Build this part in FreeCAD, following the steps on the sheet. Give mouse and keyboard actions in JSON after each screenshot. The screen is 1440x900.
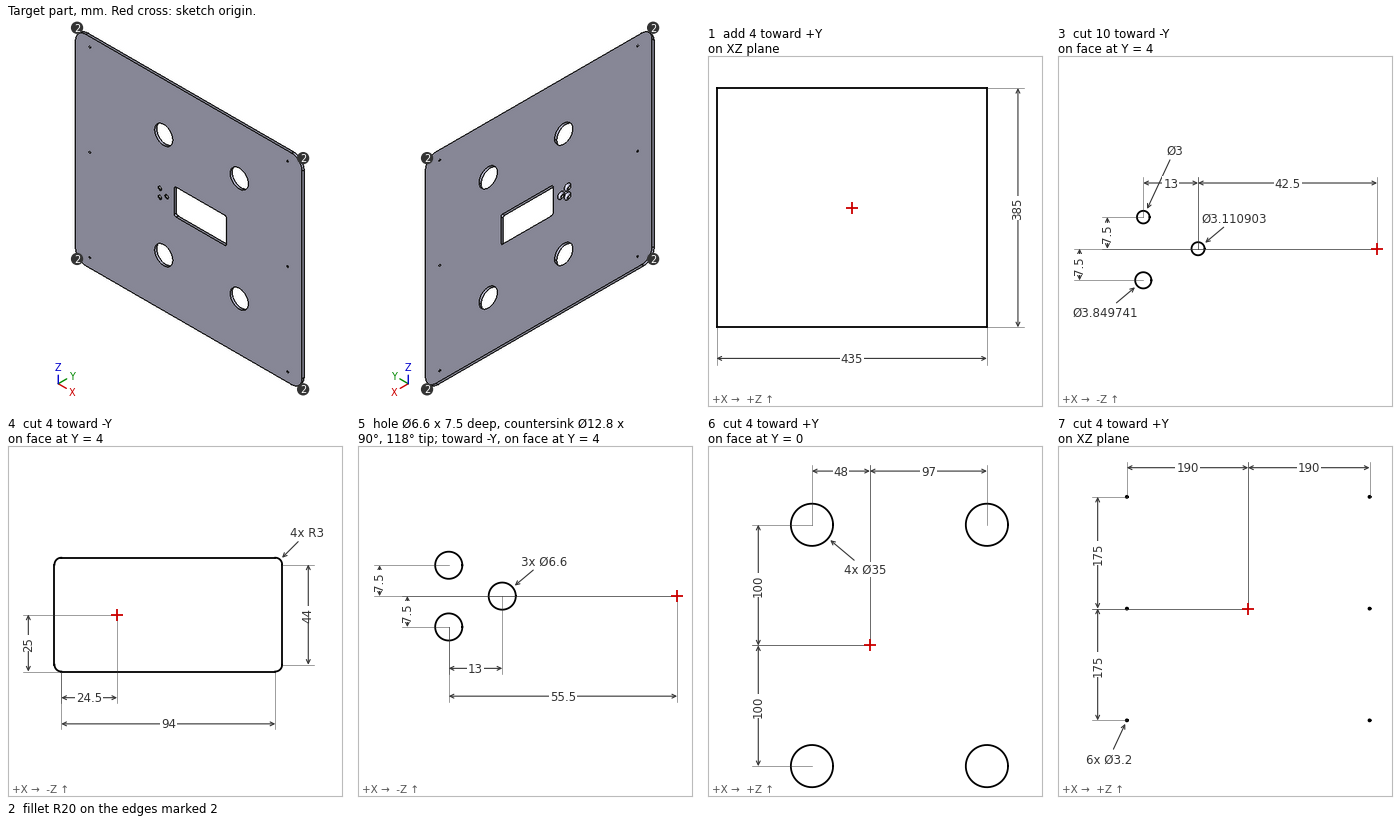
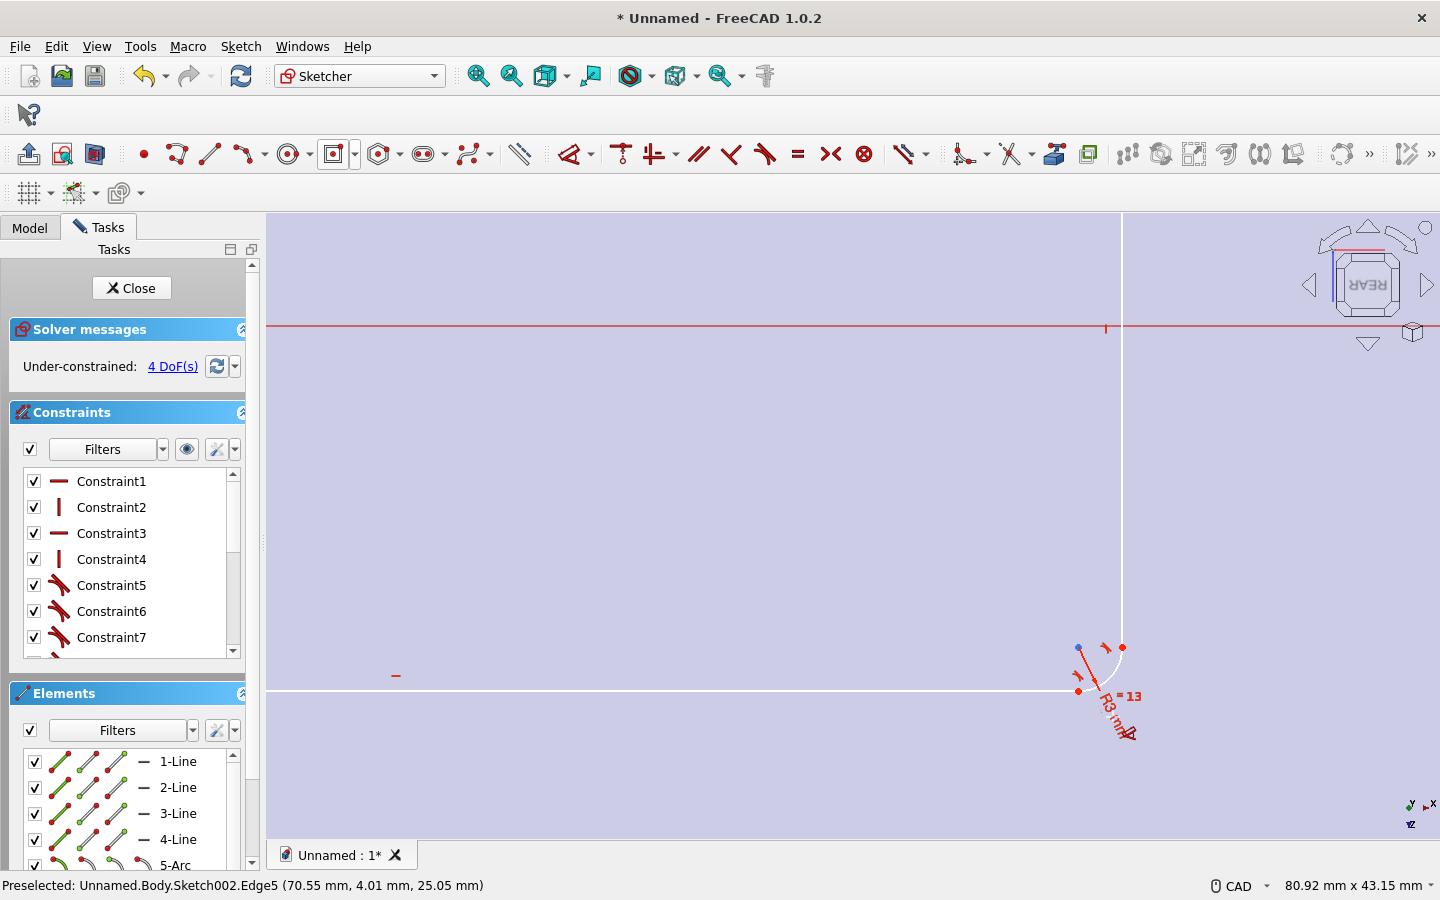
{"action": "left_click", "coordinate": [670, 691]}
{"action": "left_click", "coordinate": [686, 725]}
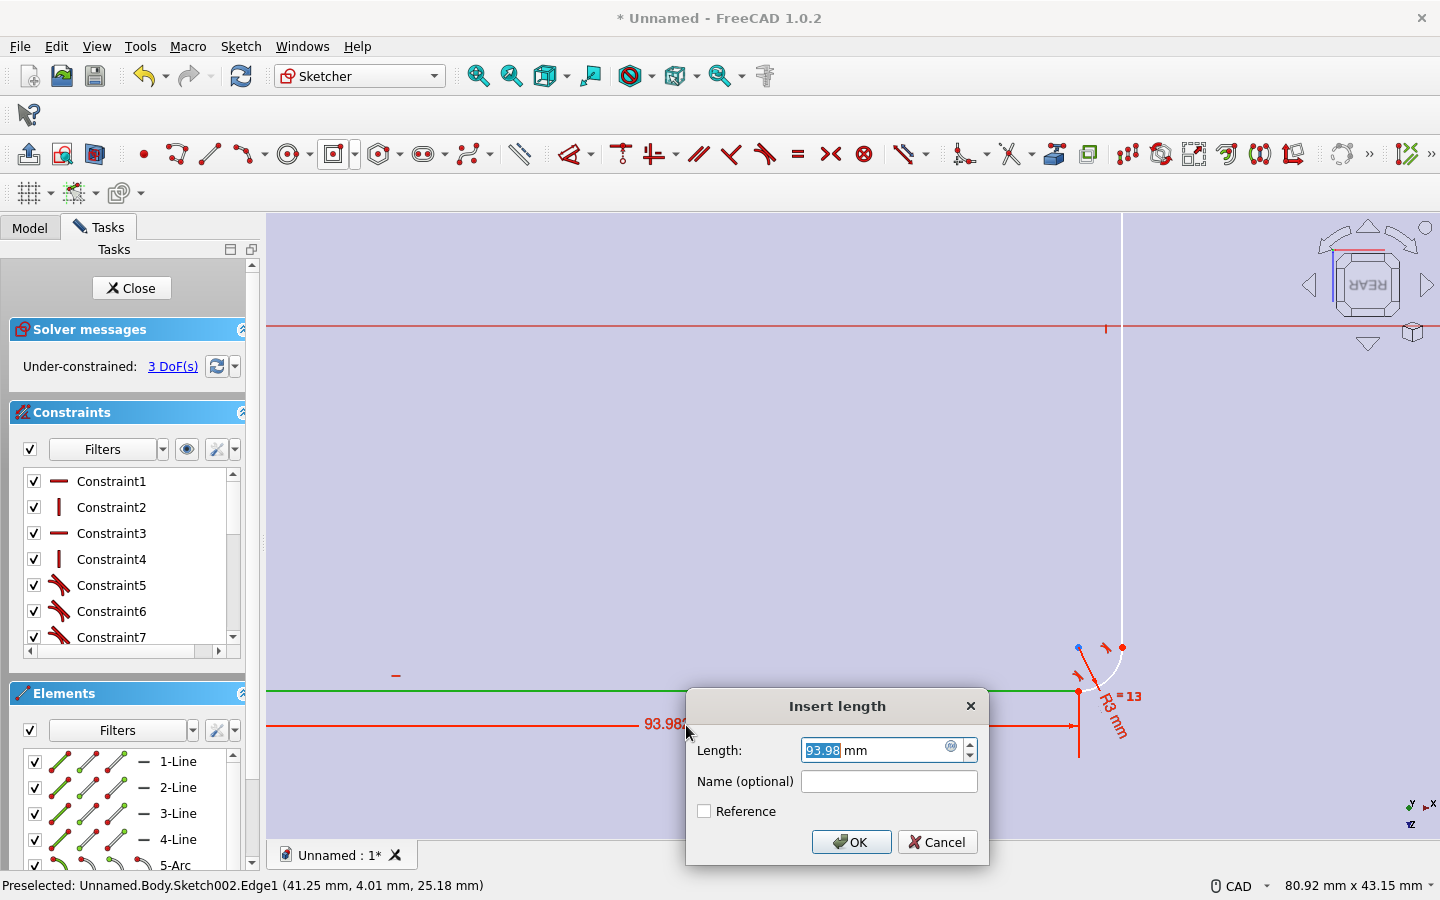
{"action": "type", "text": "94"}
{"action": "key", "text": "Return"}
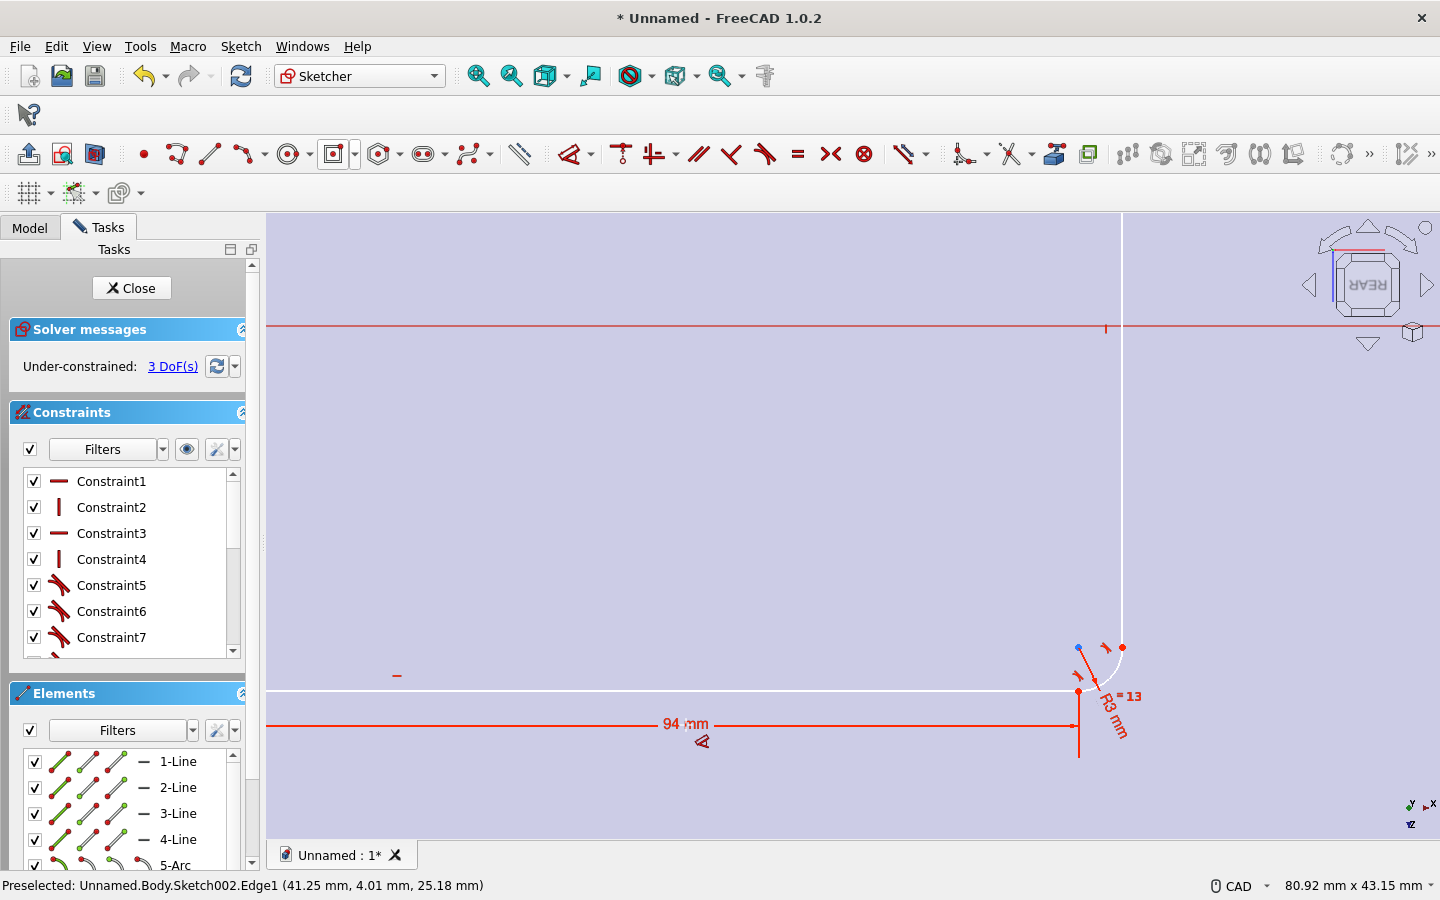
{"action": "left_click", "coordinate": [1122, 456]}
{"action": "left_click", "coordinate": [1156, 444]}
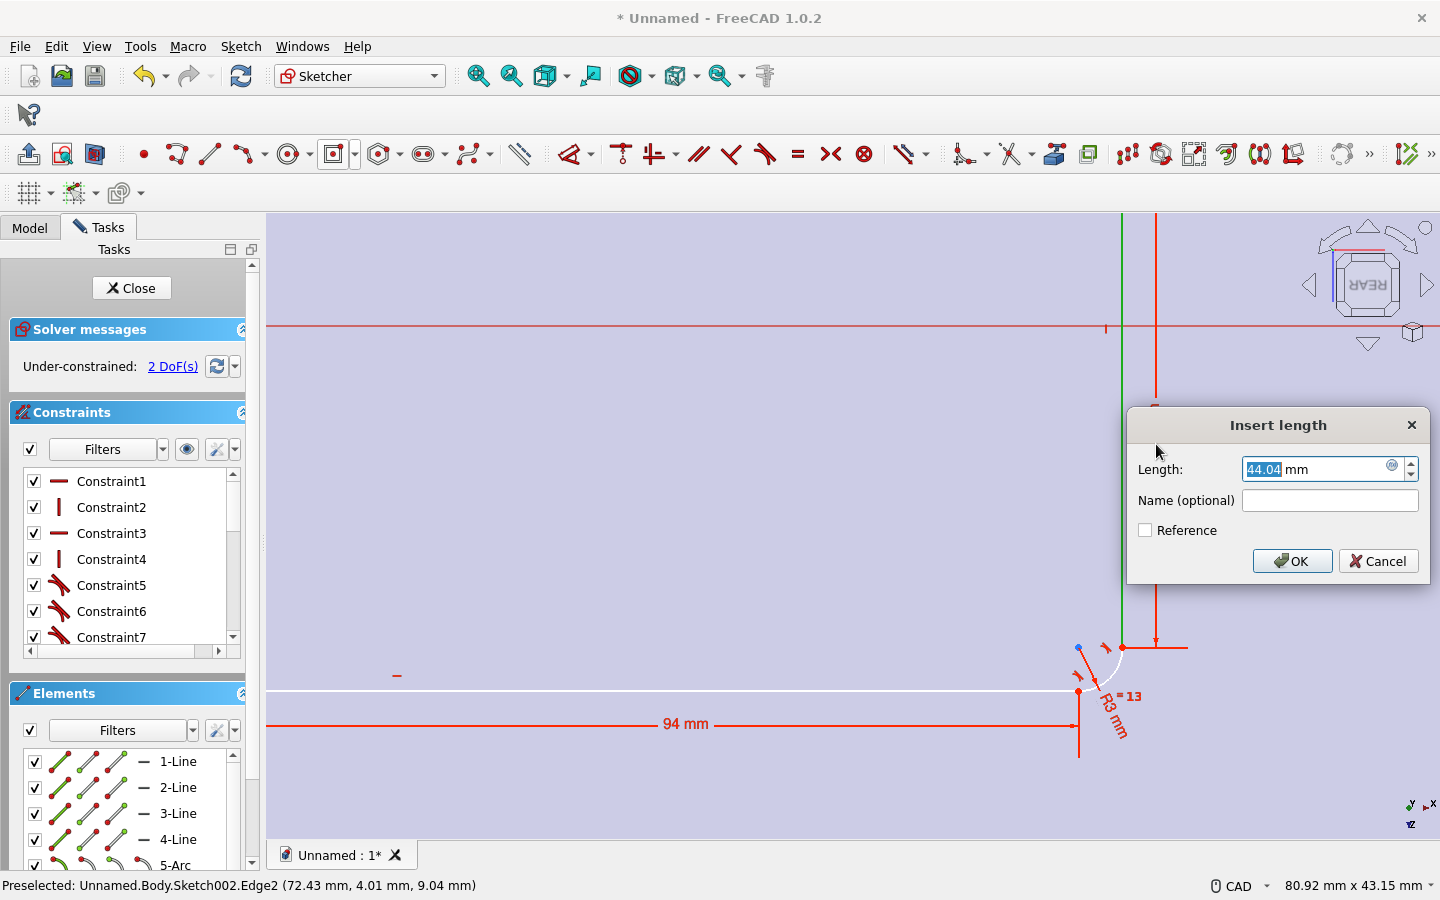
{"action": "type", "text": "44"}
{"action": "key", "text": "Return"}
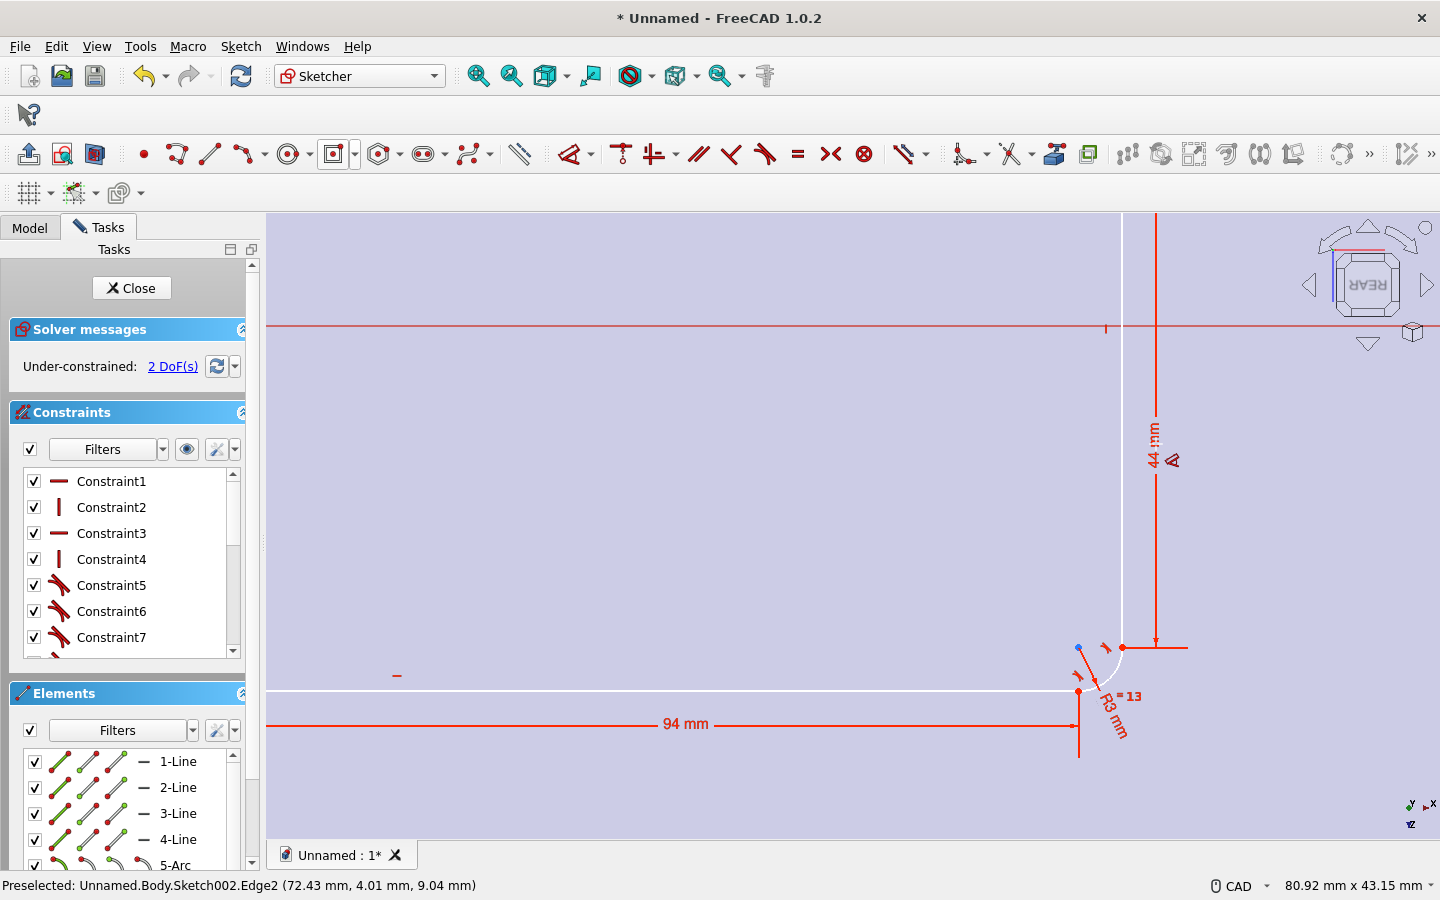
{"action": "scroll", "coordinate": [1100, 689], "scroll_direction": "down", "scroll_amount": 4}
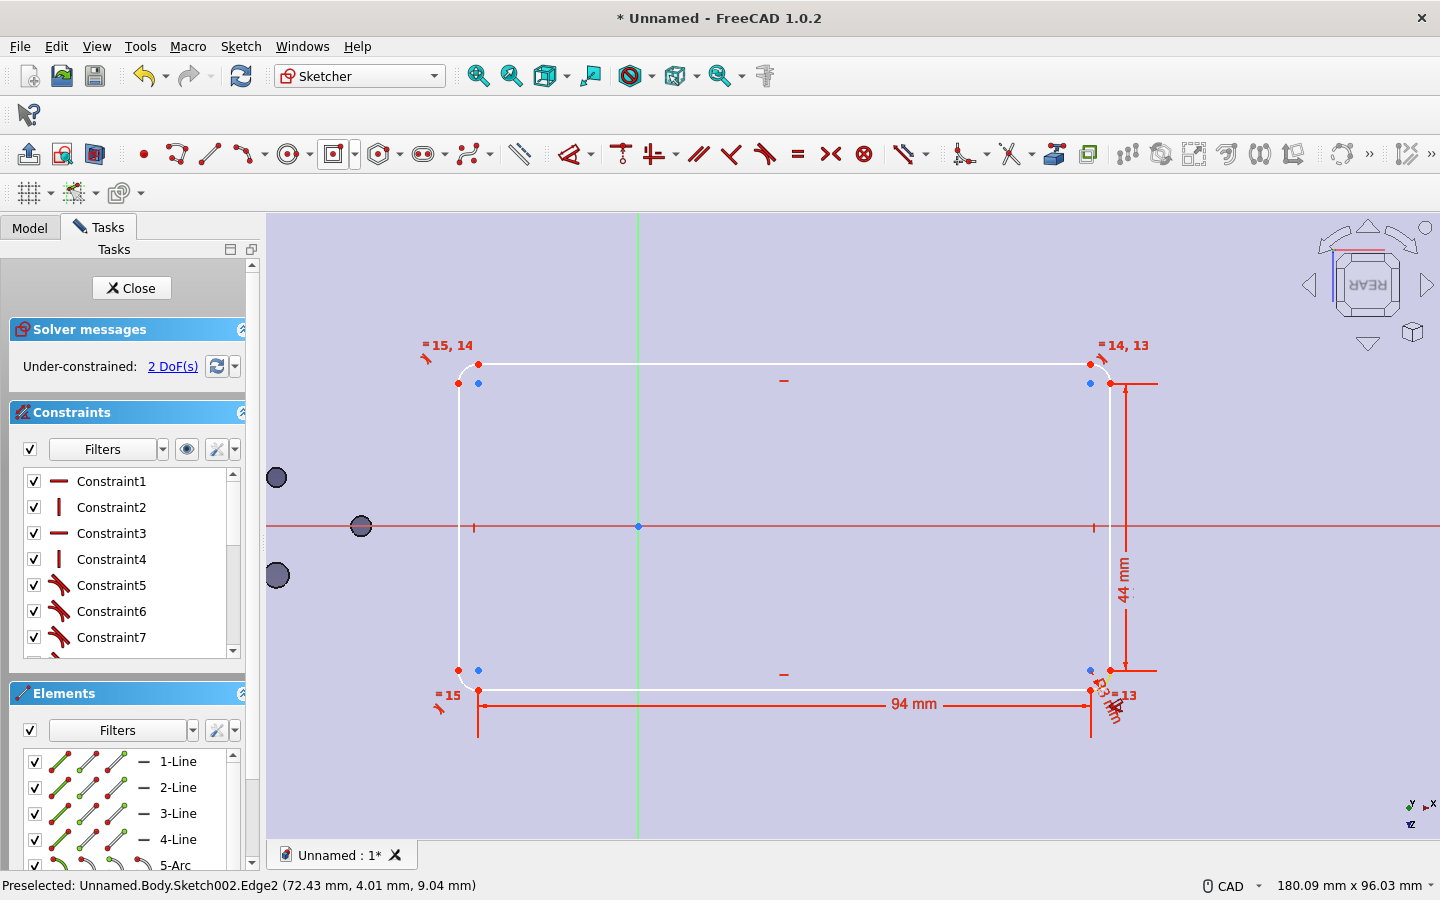
{"action": "left_click", "coordinate": [478, 690]}
{"action": "left_click", "coordinate": [444, 608]}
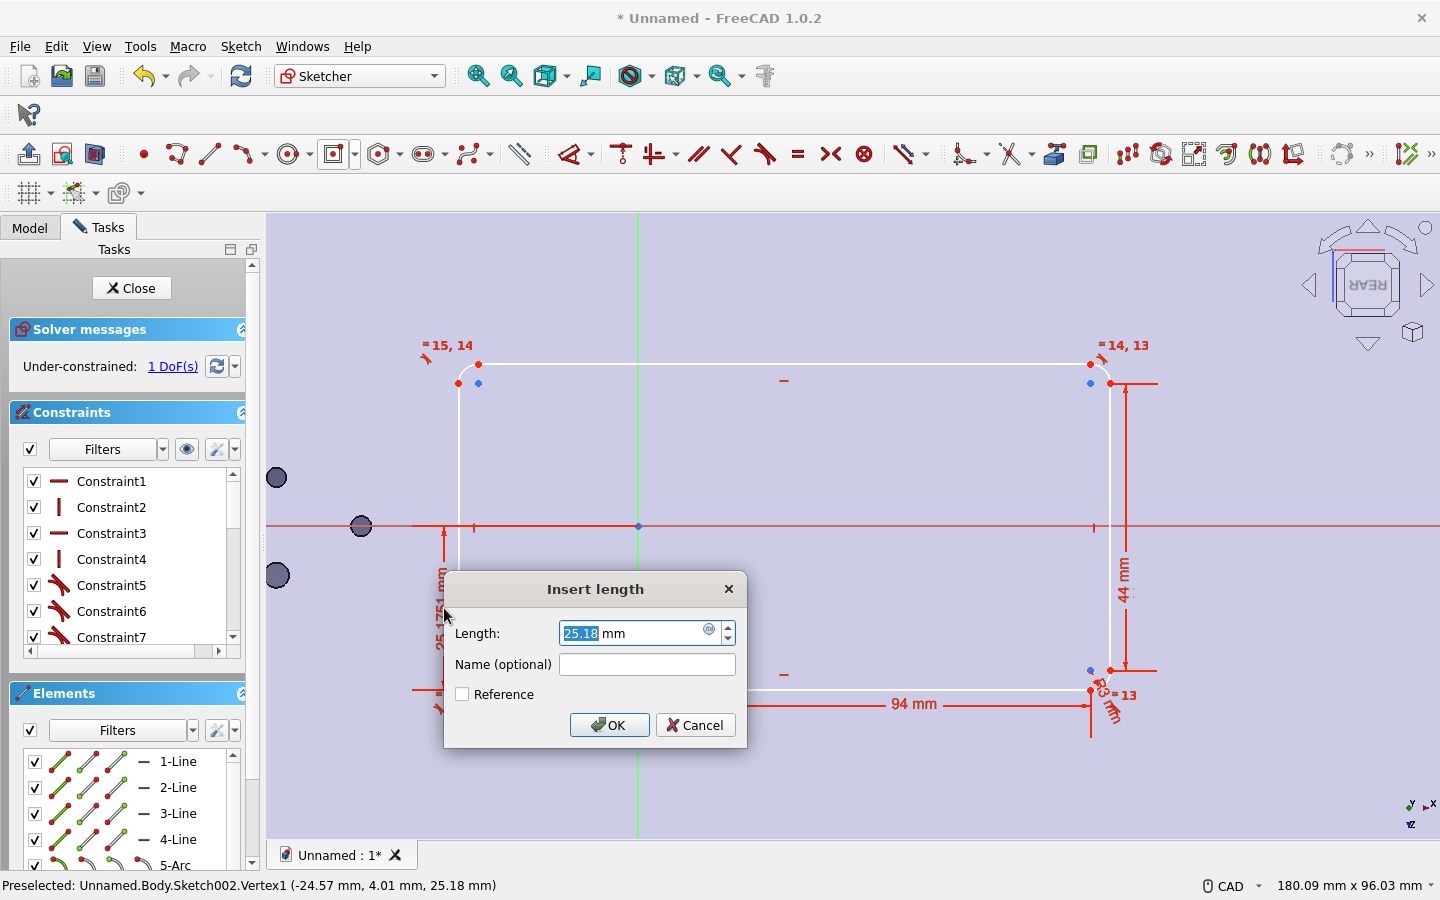
{"action": "type", "text": "25"}
{"action": "key", "text": "Return"}